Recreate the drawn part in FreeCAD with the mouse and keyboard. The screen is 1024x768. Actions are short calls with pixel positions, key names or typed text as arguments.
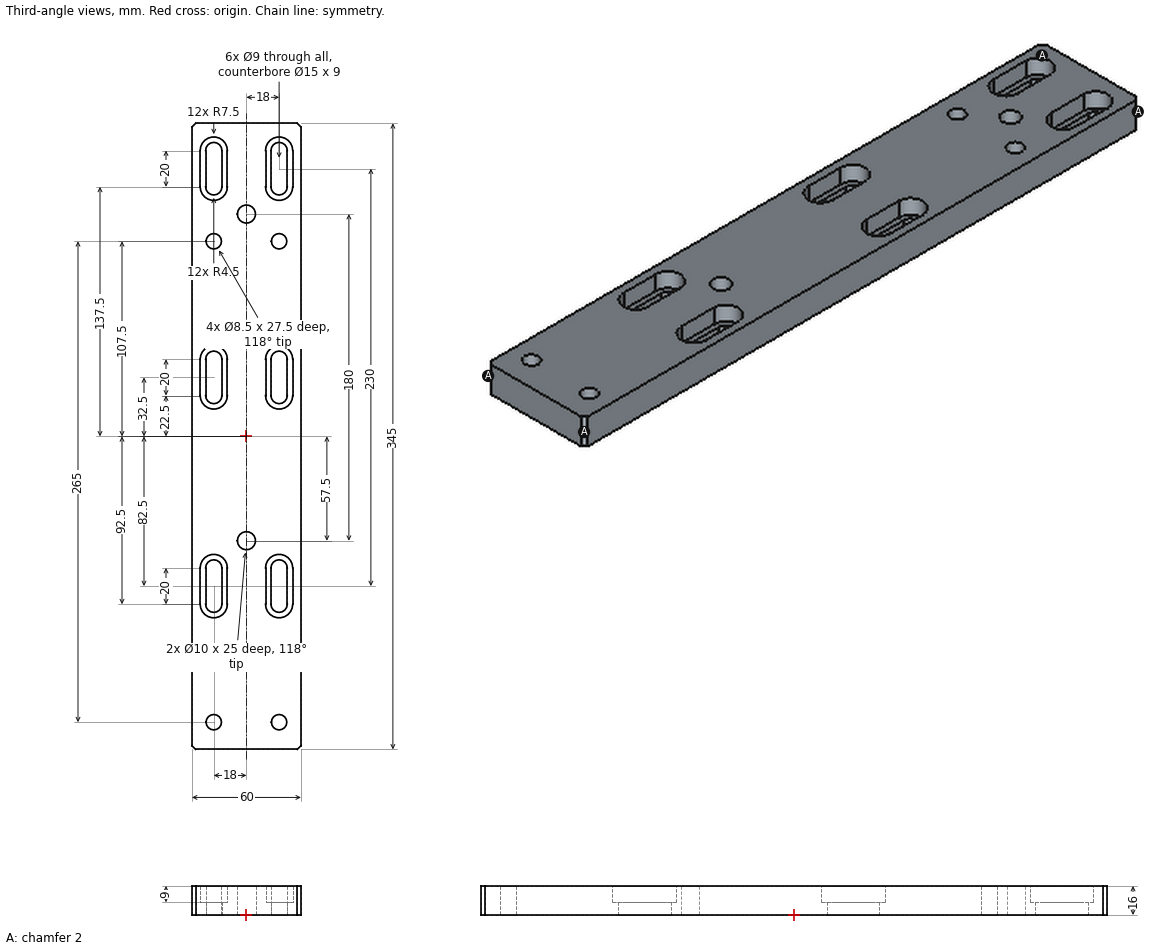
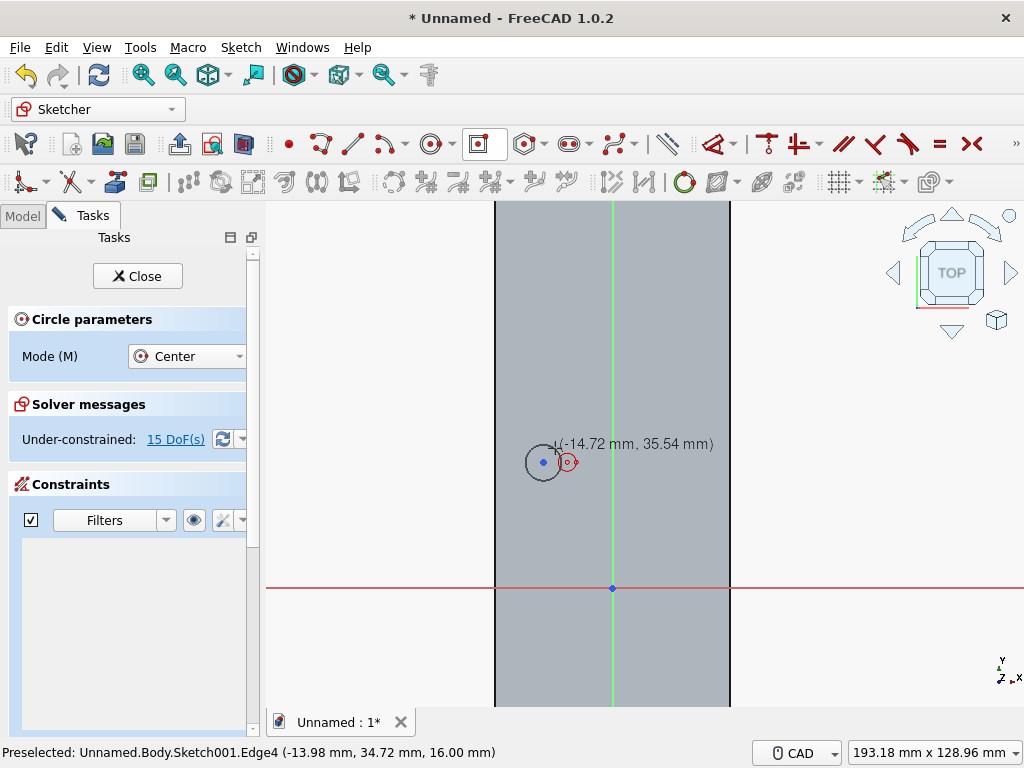
scroll(683, 461, up, 2)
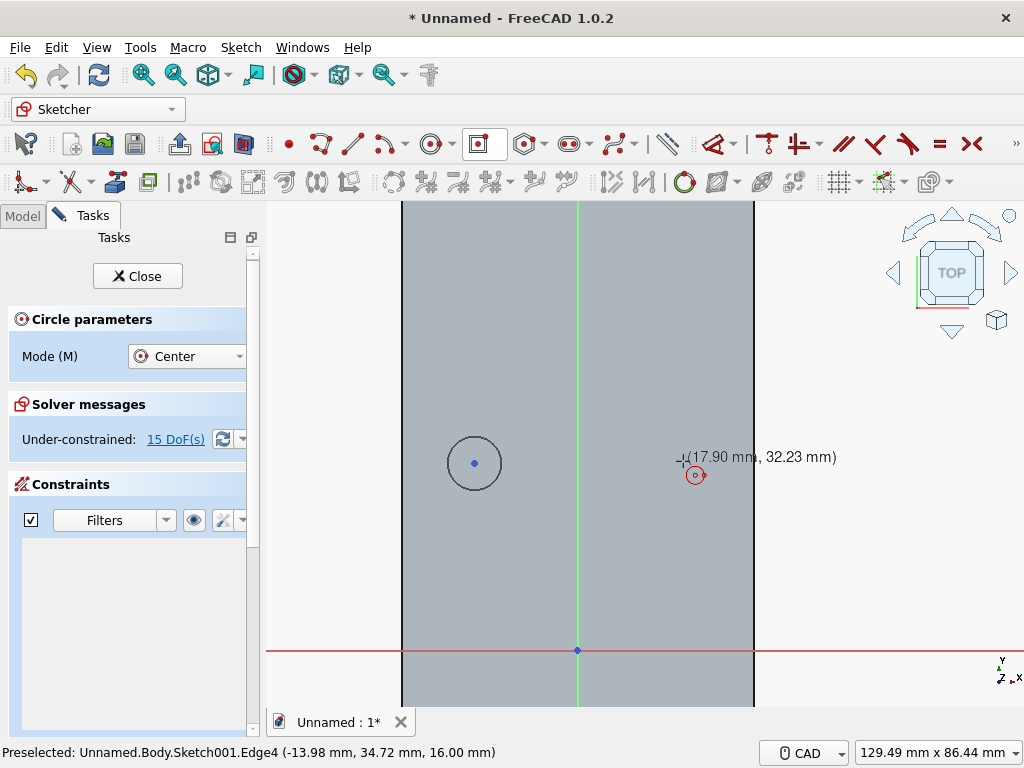
scroll(576, 452, down, 7)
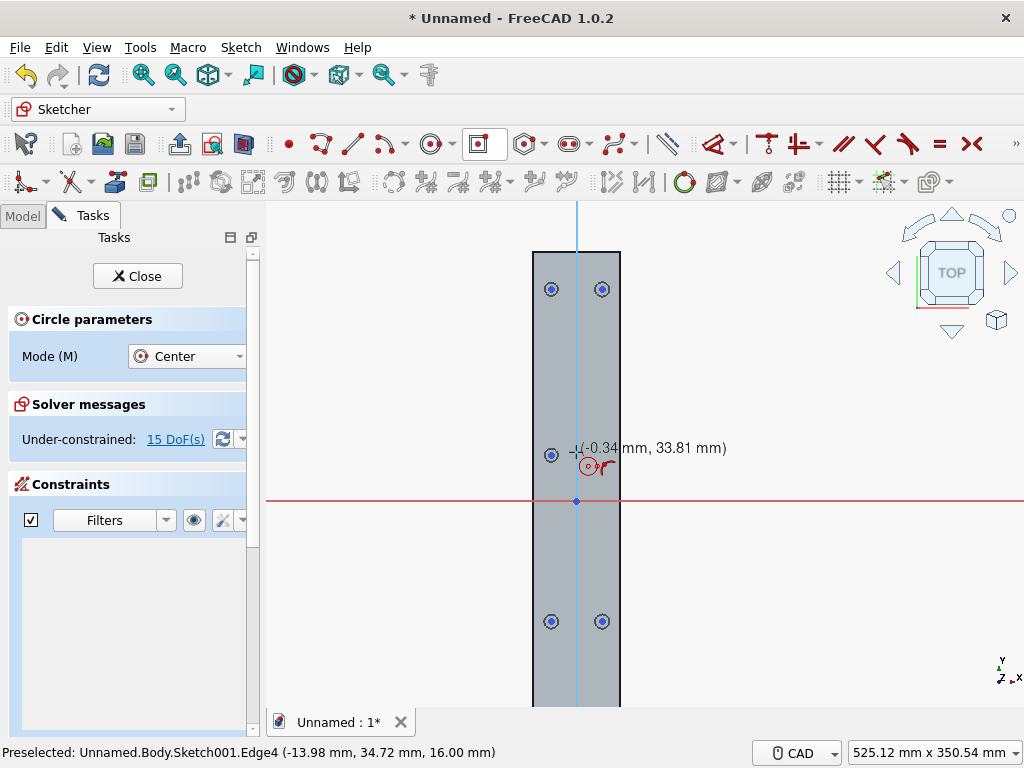
click(603, 455)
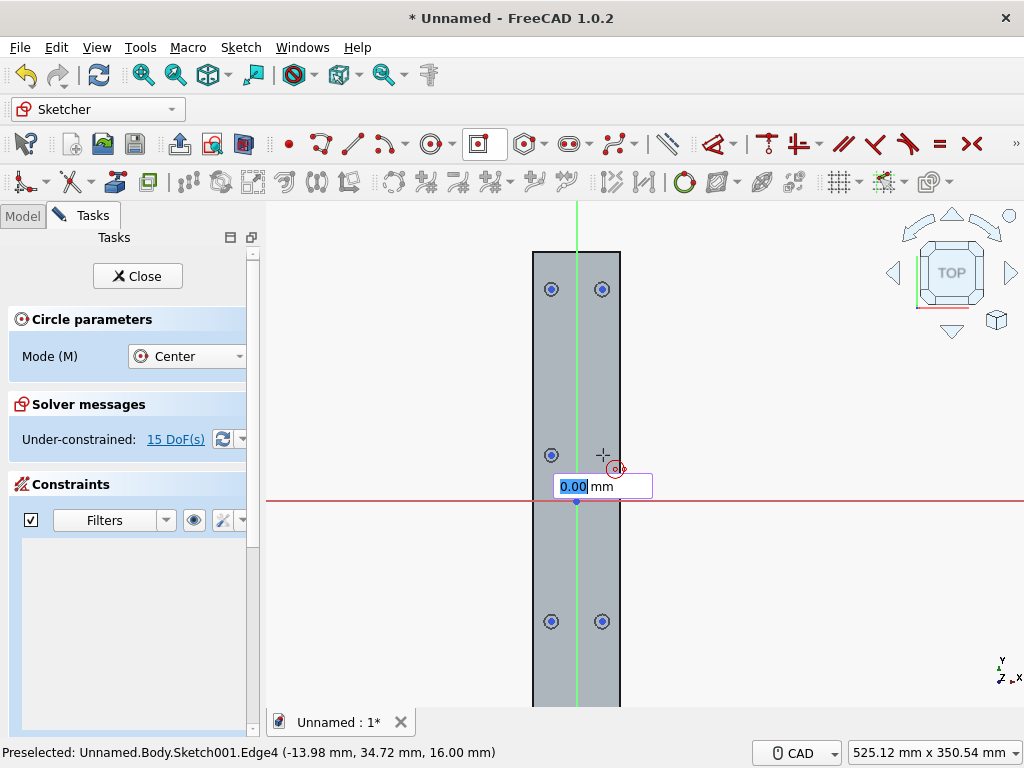
scroll(607, 450, up, 5)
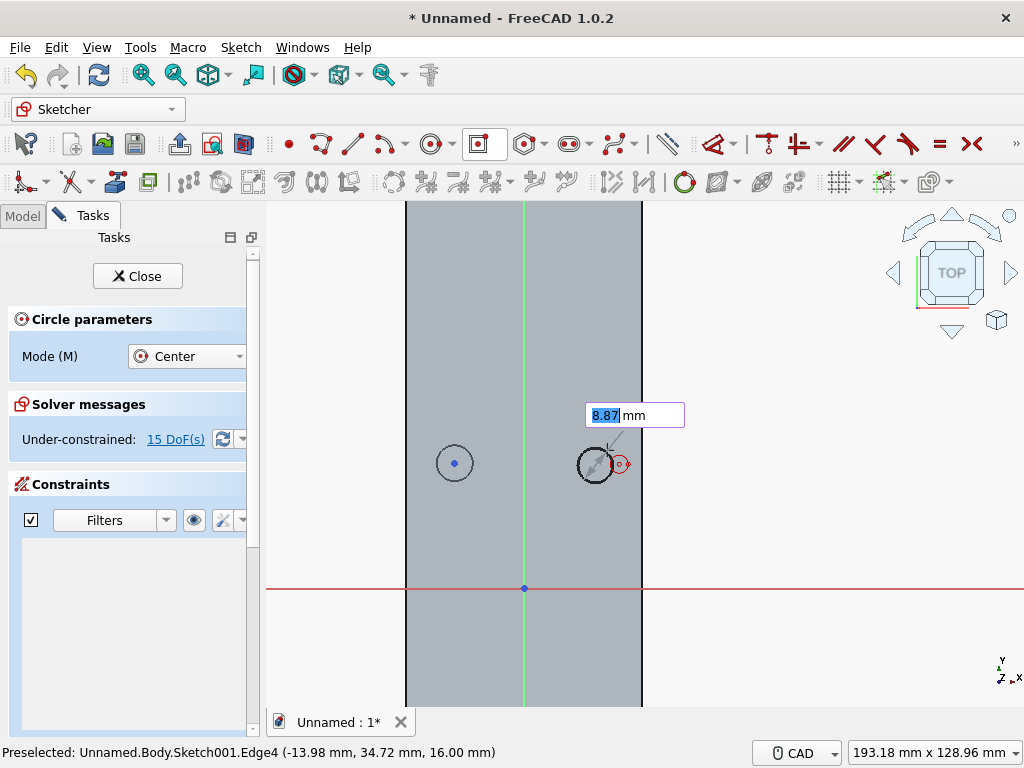
click(607, 449)
key(Escape)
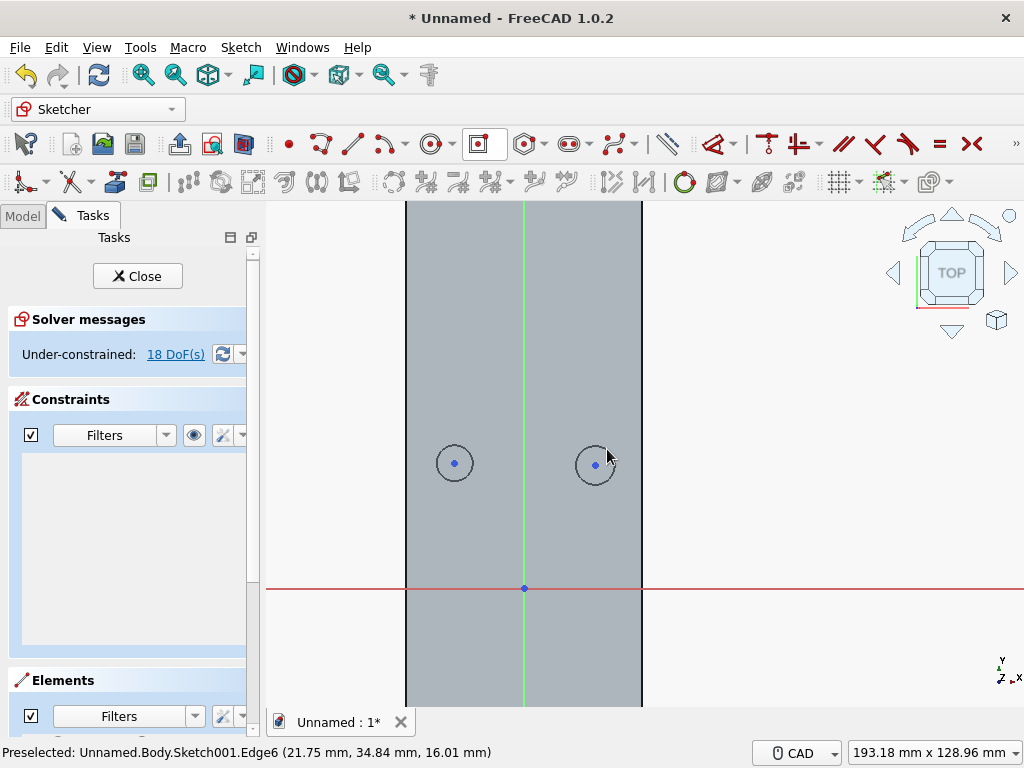
scroll(607, 450, down, 5)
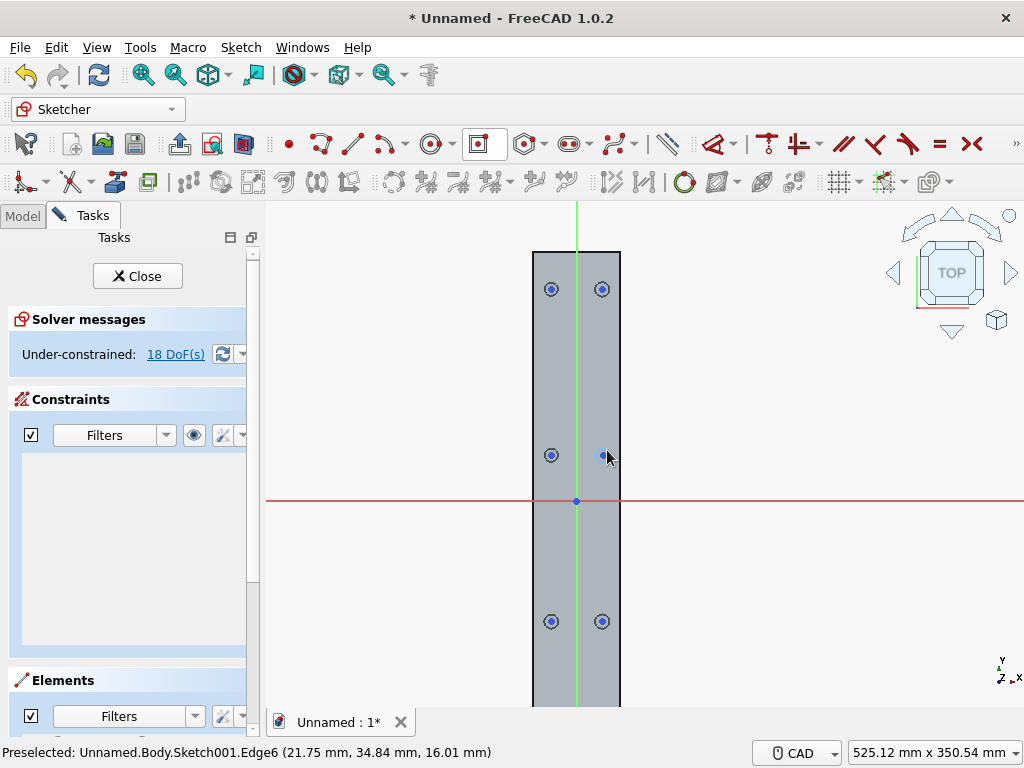
scroll(607, 284, up, 4)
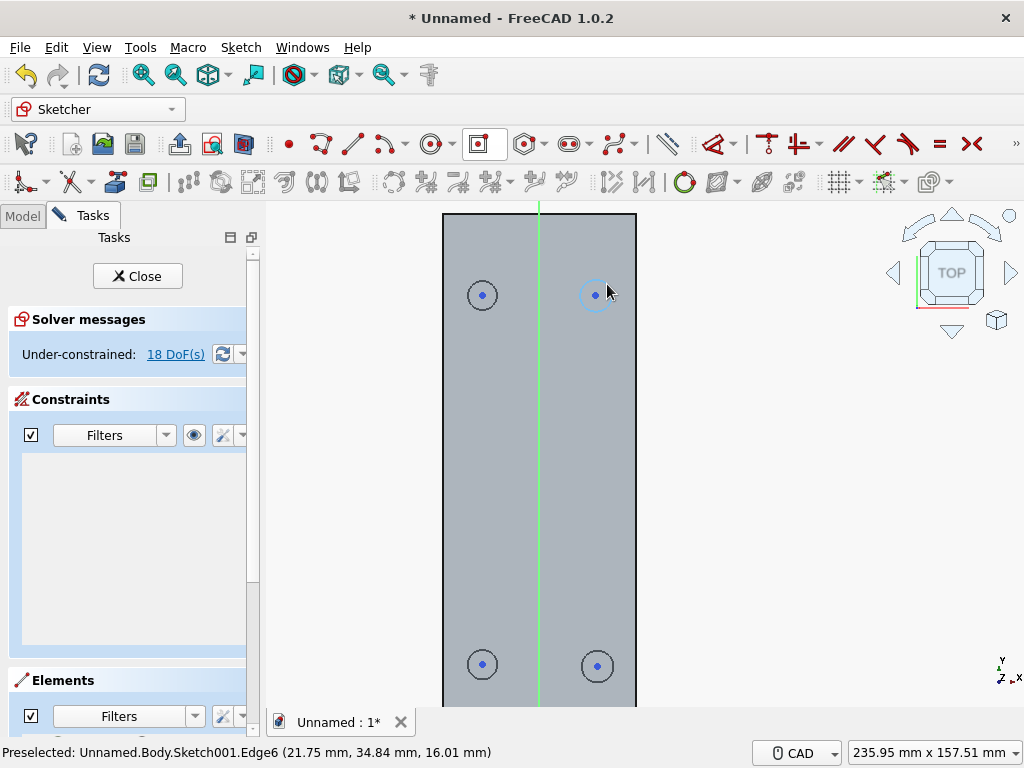
click(607, 285)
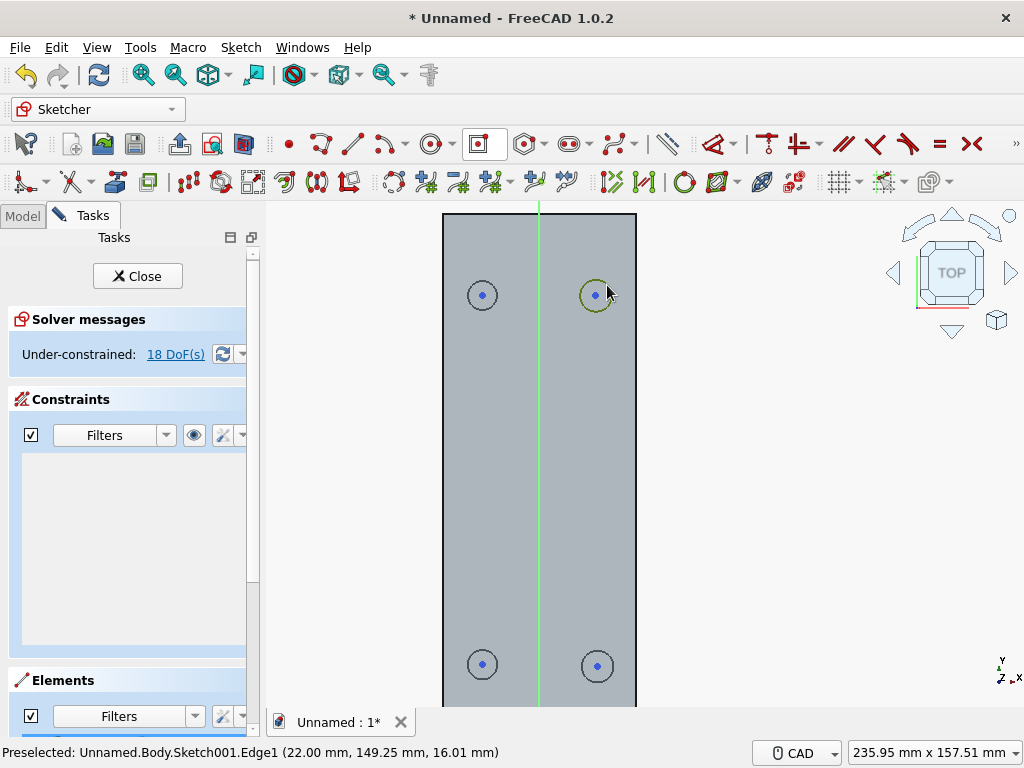
scroll(607, 283, down, 4)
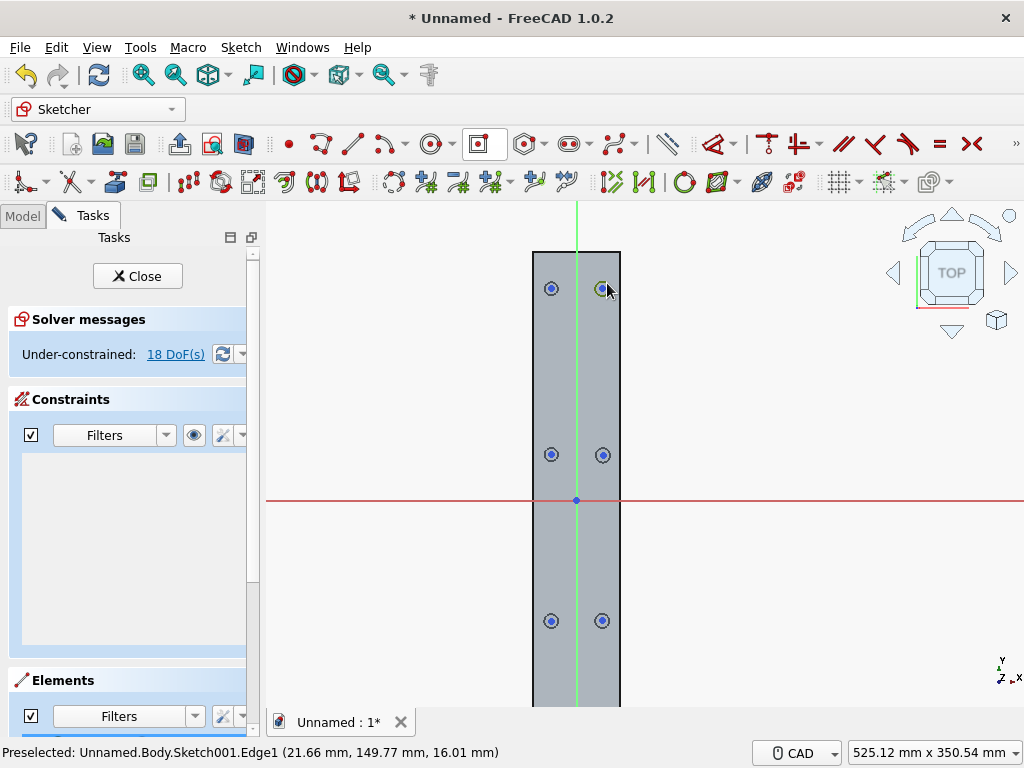
scroll(556, 616, up, 4)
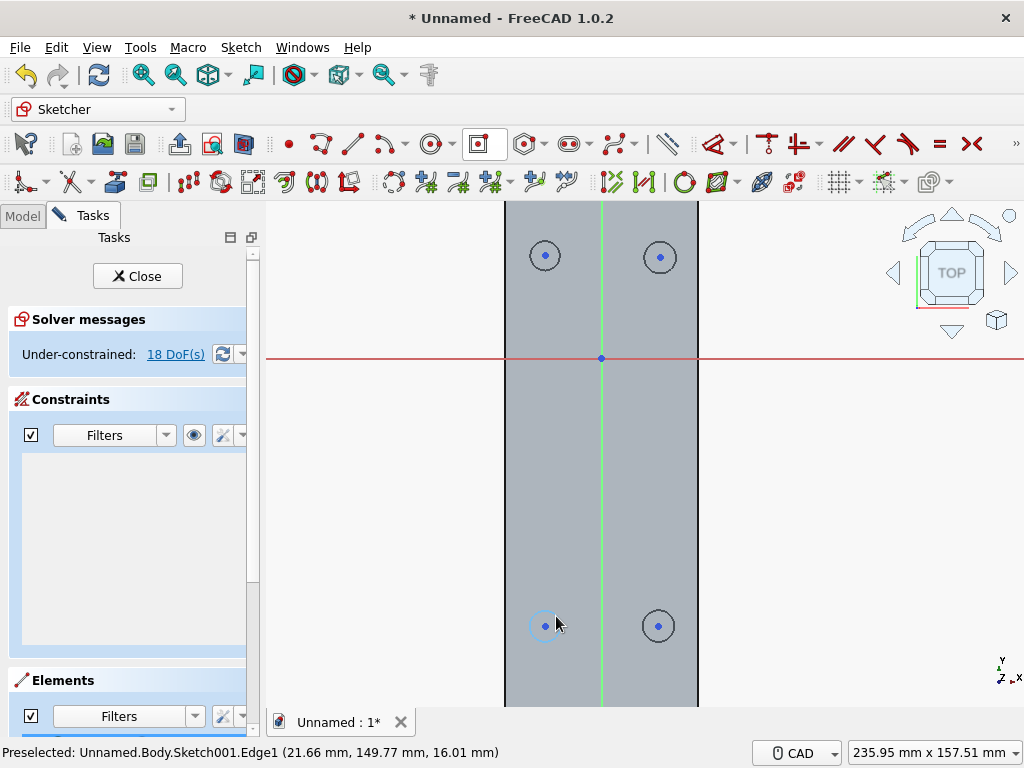
click(556, 615)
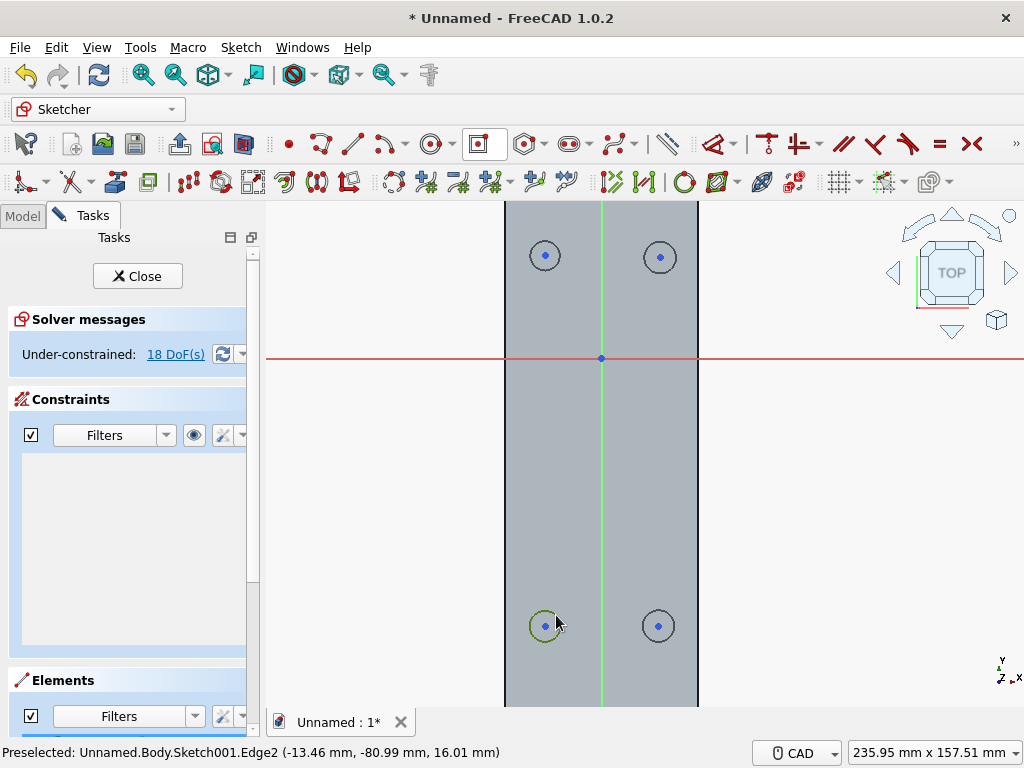
scroll(556, 617, down, 4)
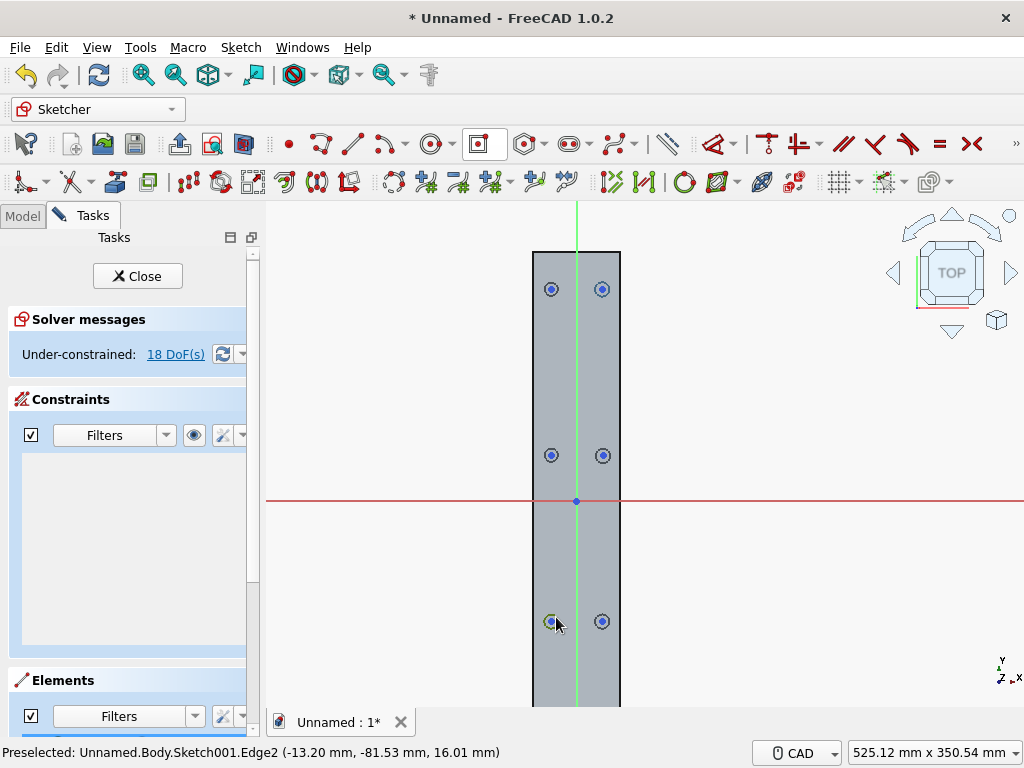
scroll(556, 285, up, 4)